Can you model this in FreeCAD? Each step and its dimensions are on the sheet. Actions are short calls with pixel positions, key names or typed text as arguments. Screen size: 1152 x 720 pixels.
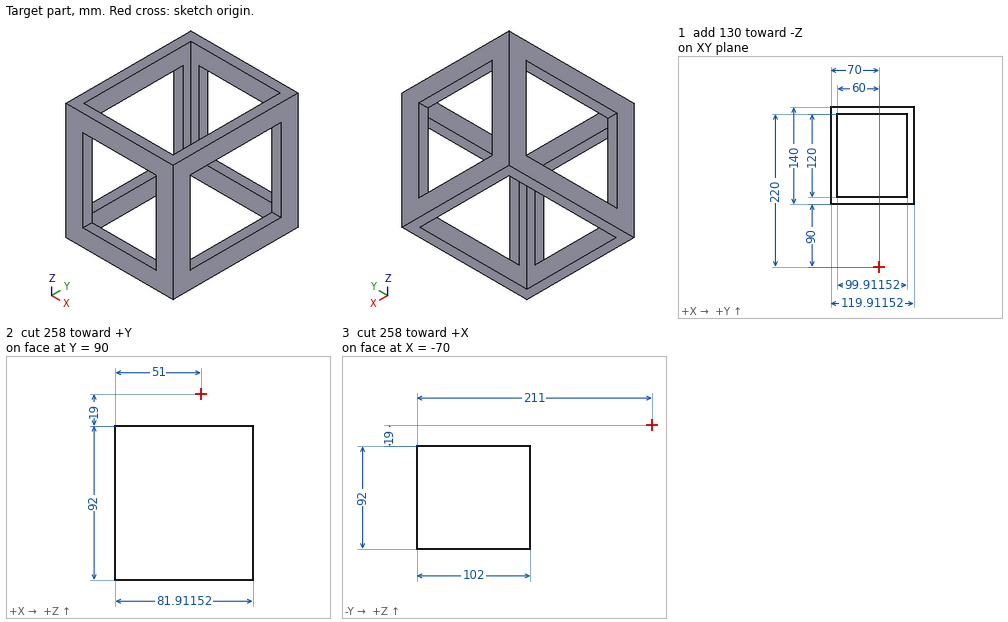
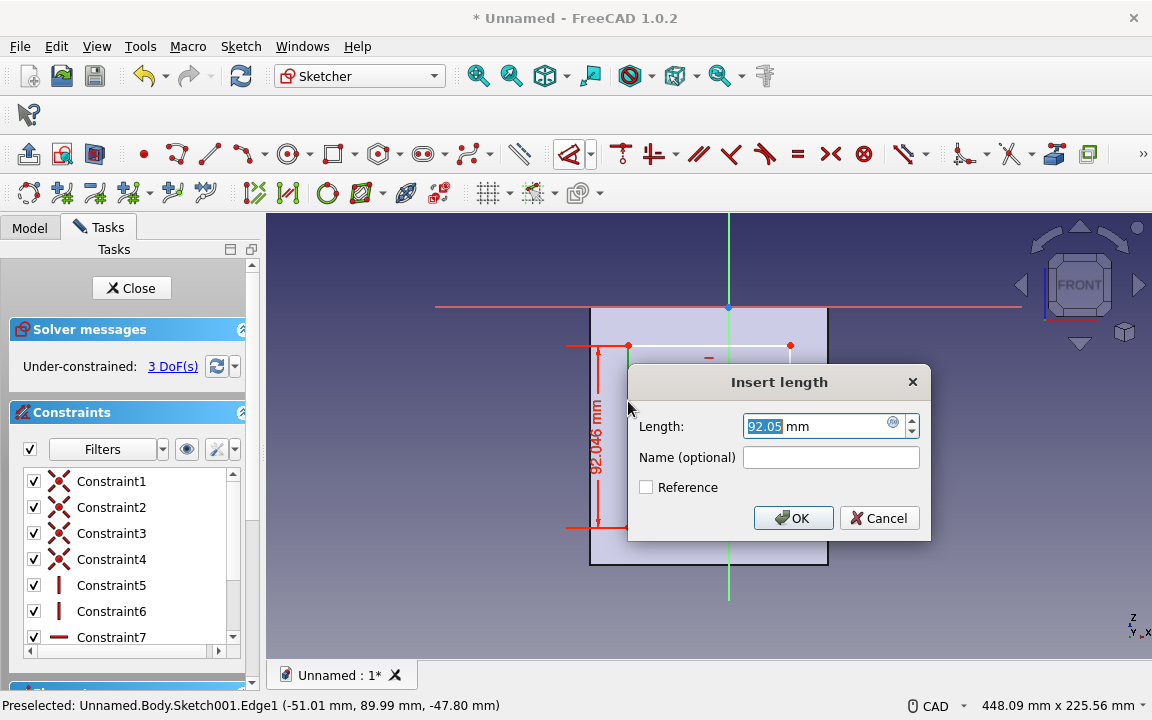
text(92)
key(Return)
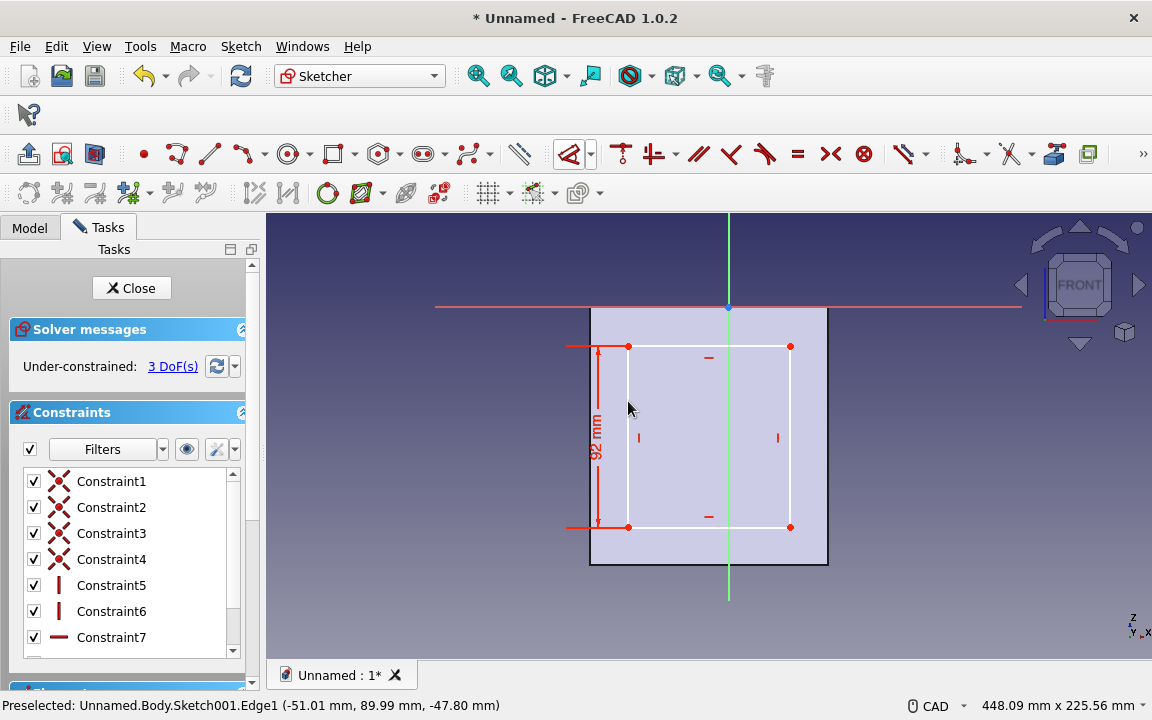
click(628, 346)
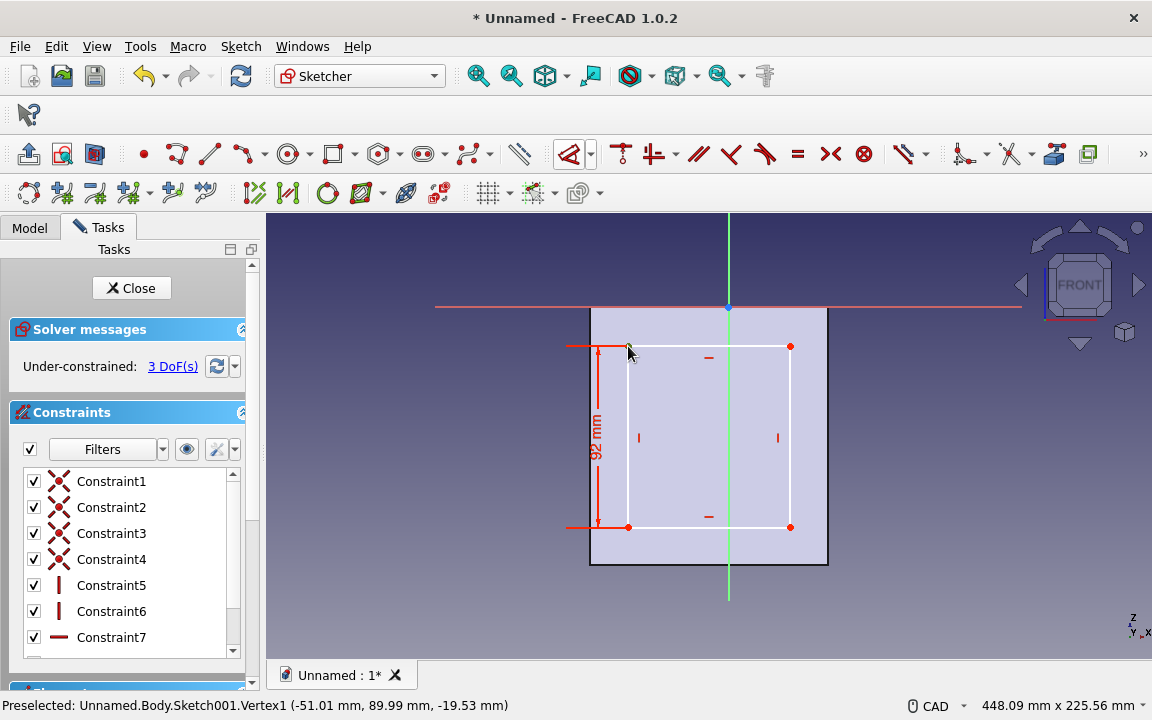
key(l)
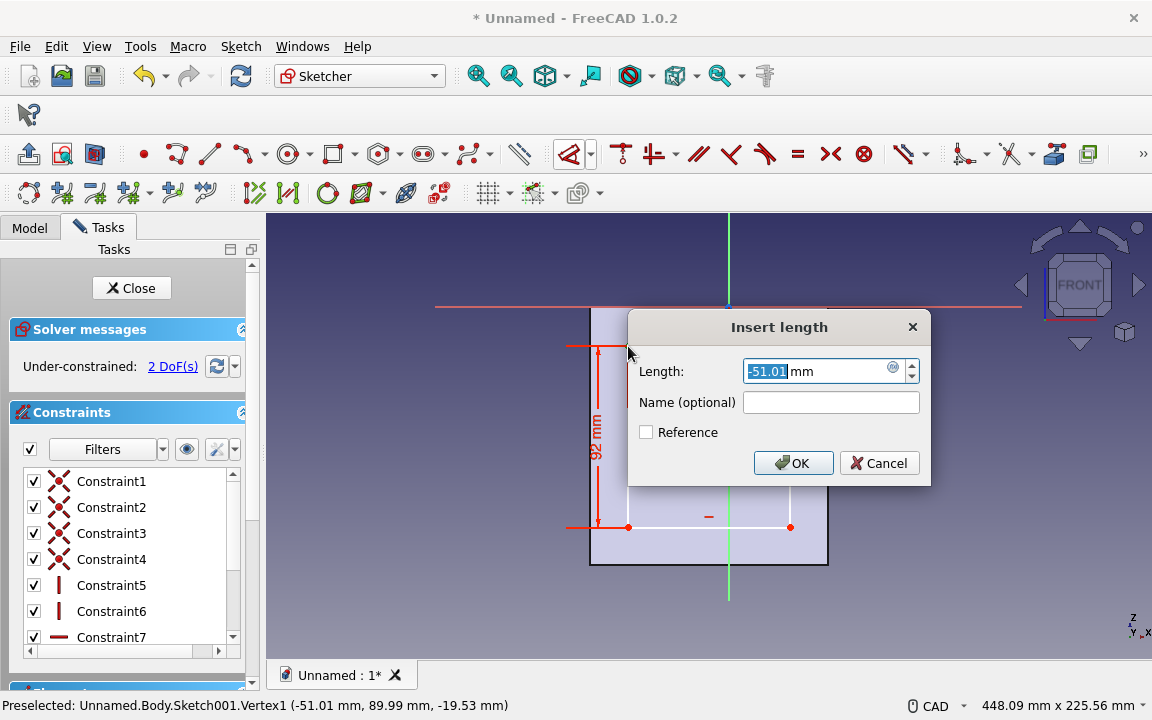
text(-51)
key(Return)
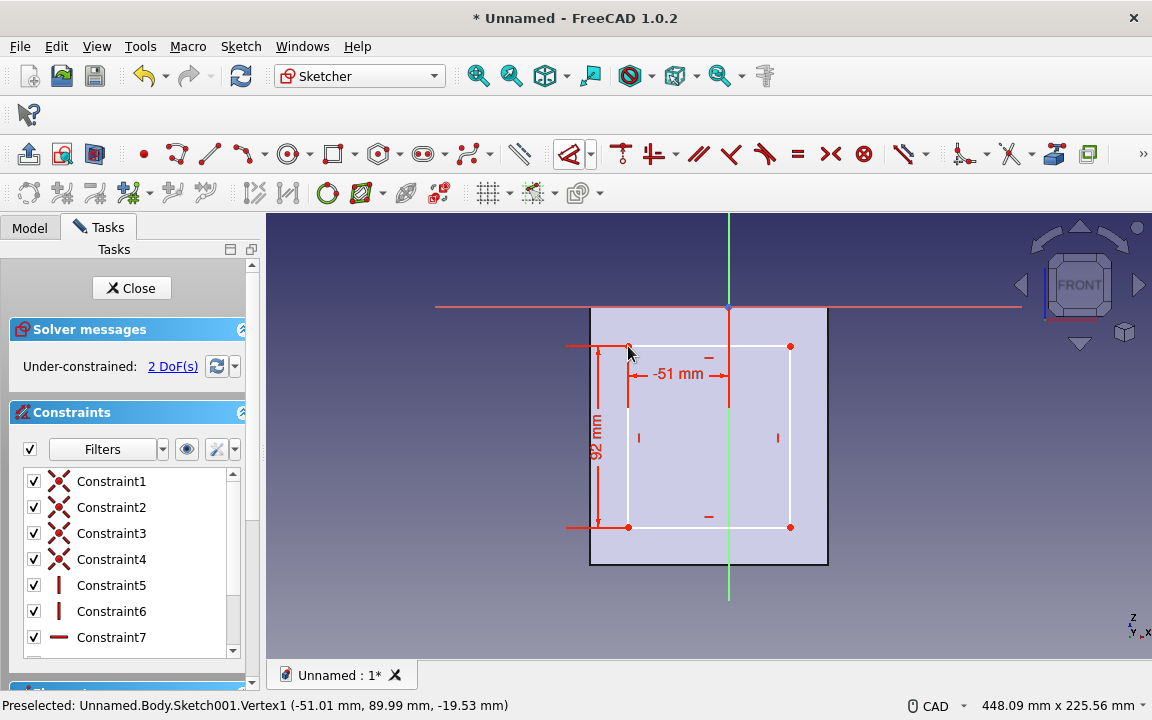
click(628, 346)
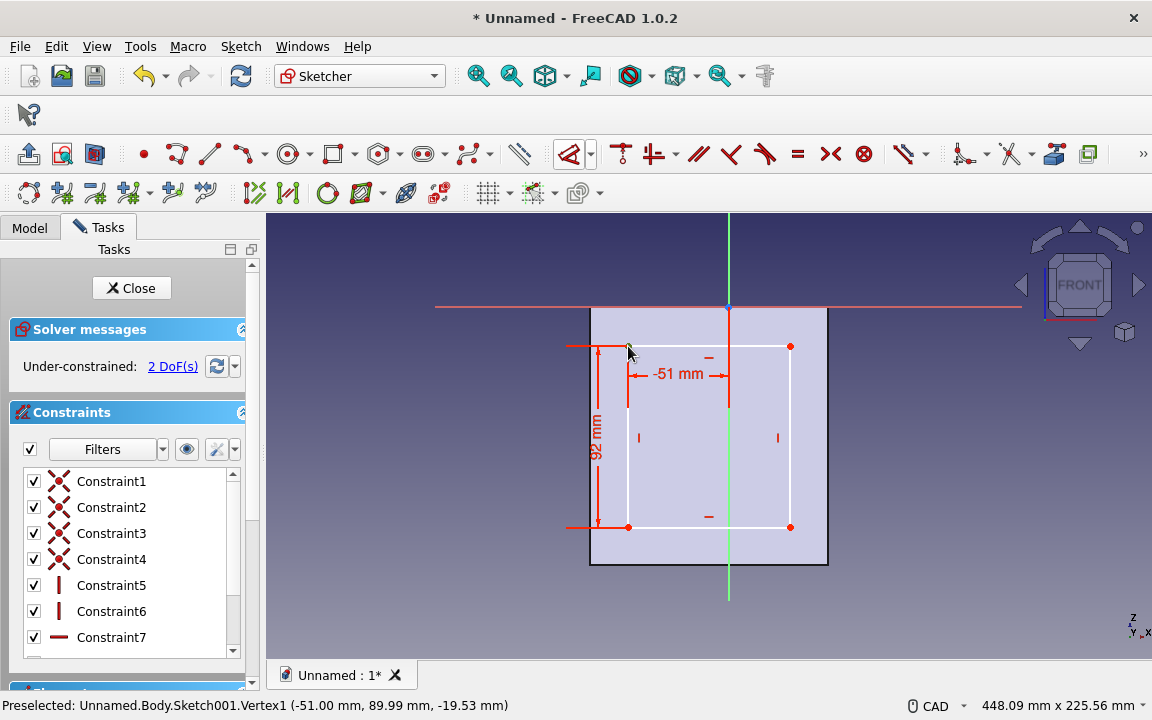
key(i)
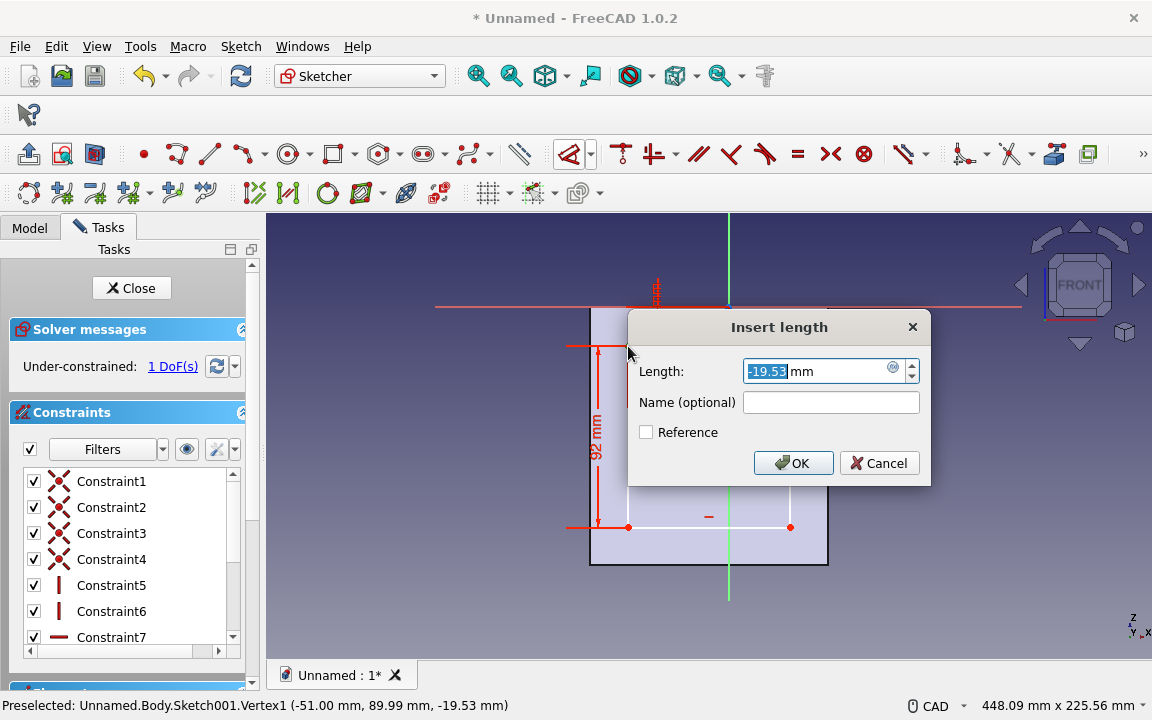
text(-19)
key(Return)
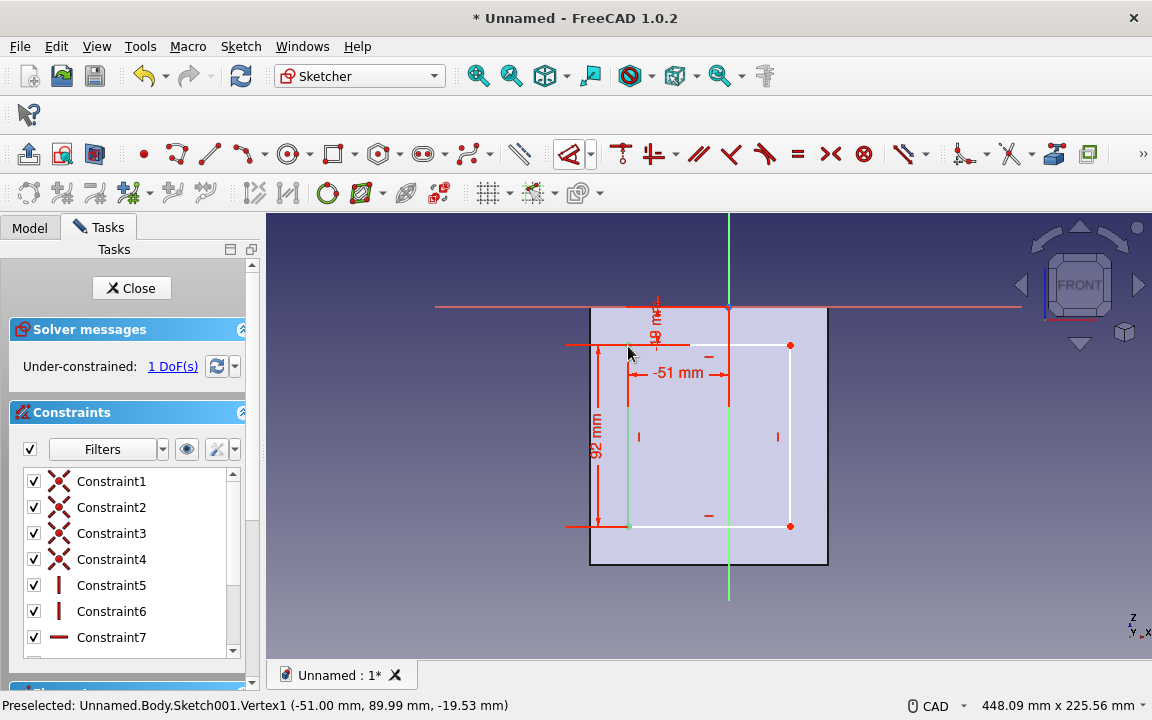
click(677, 527)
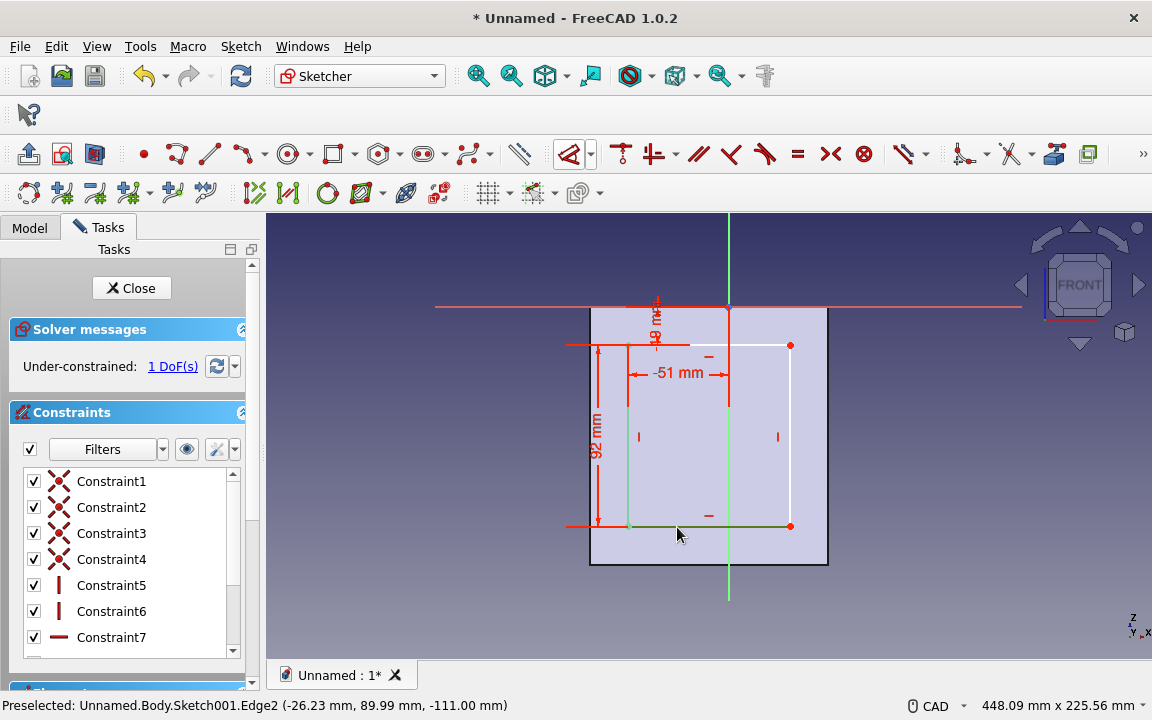
key(l)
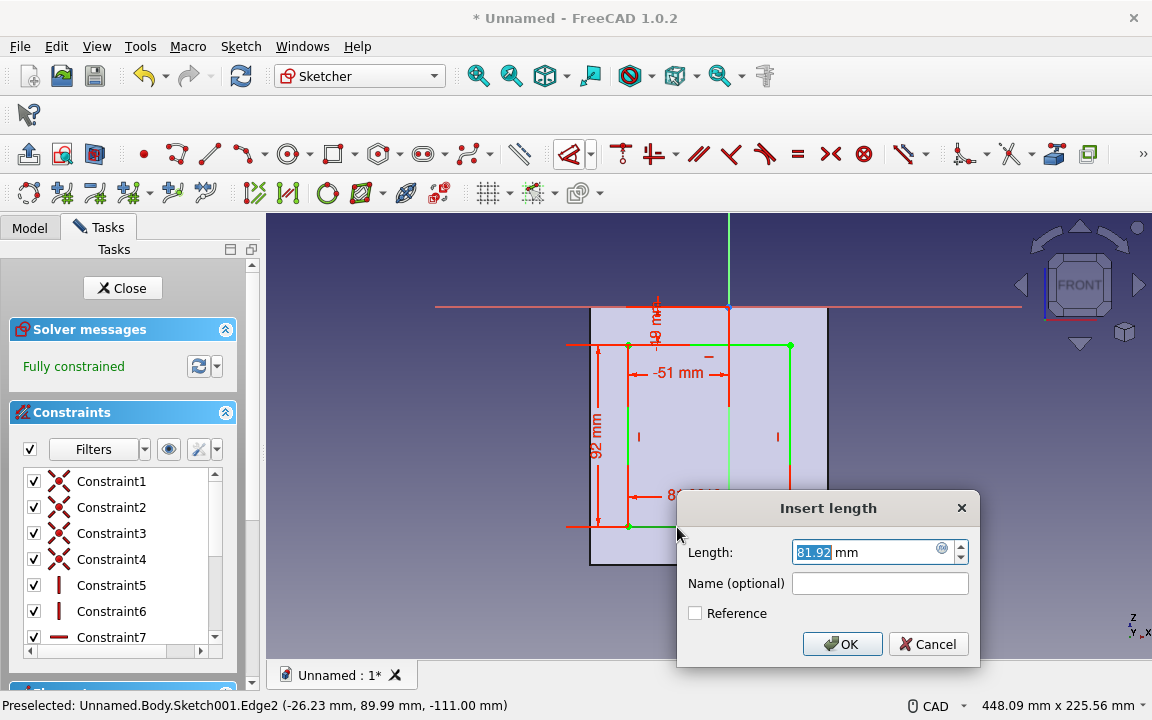
text(81.91152)
key(Return)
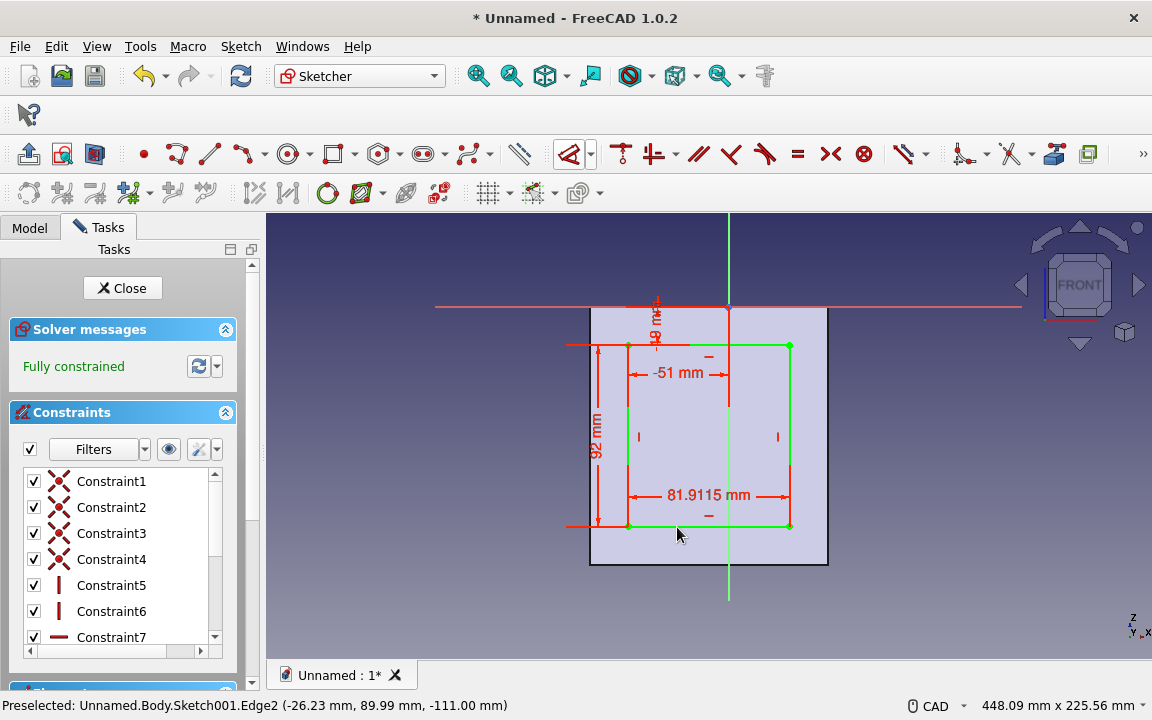
click(123, 288)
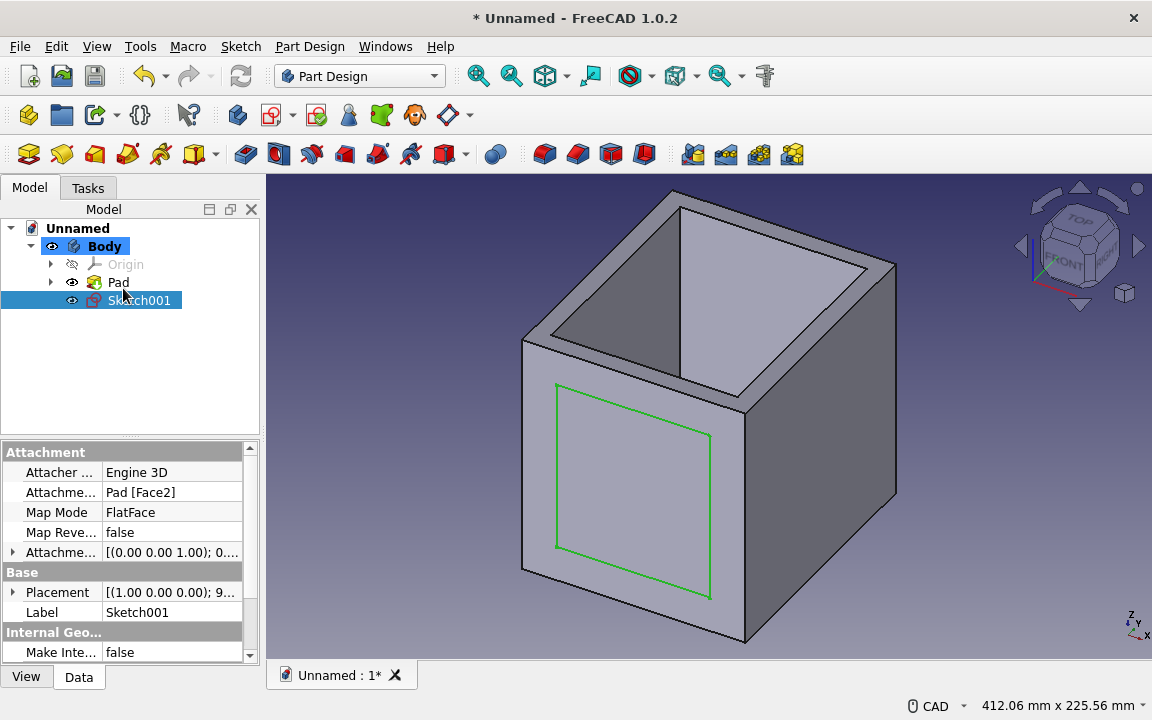
click(246, 154)